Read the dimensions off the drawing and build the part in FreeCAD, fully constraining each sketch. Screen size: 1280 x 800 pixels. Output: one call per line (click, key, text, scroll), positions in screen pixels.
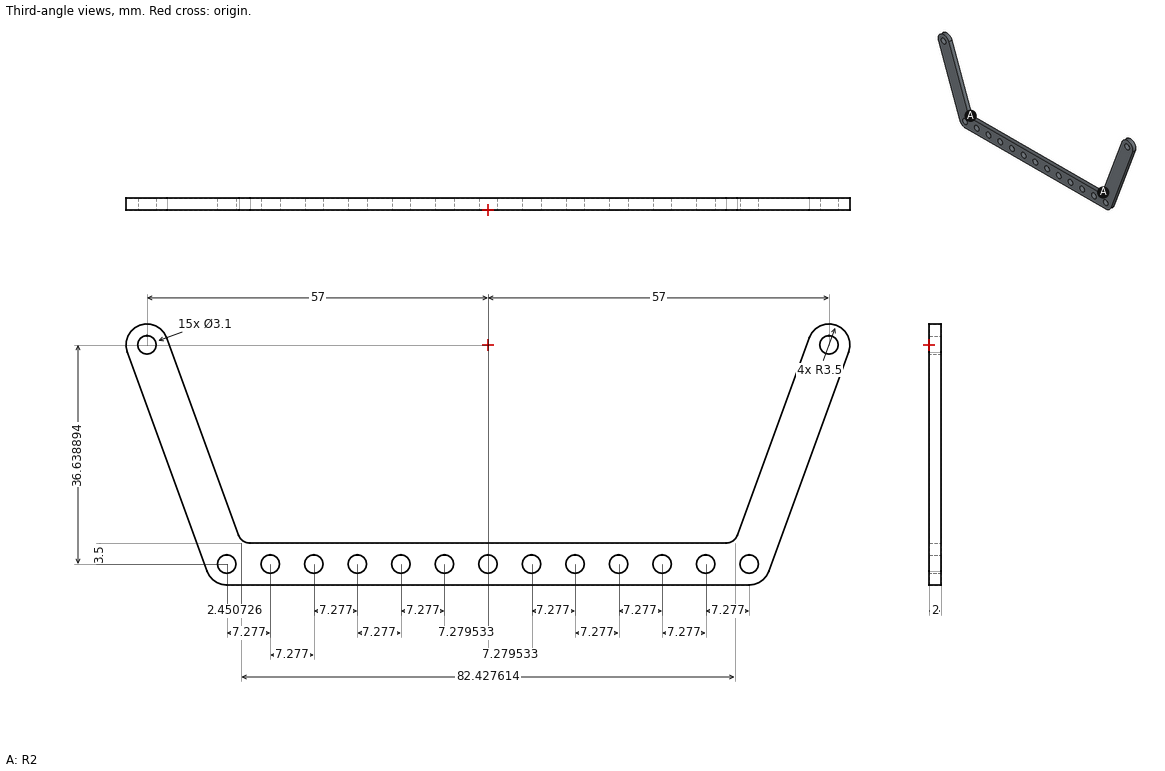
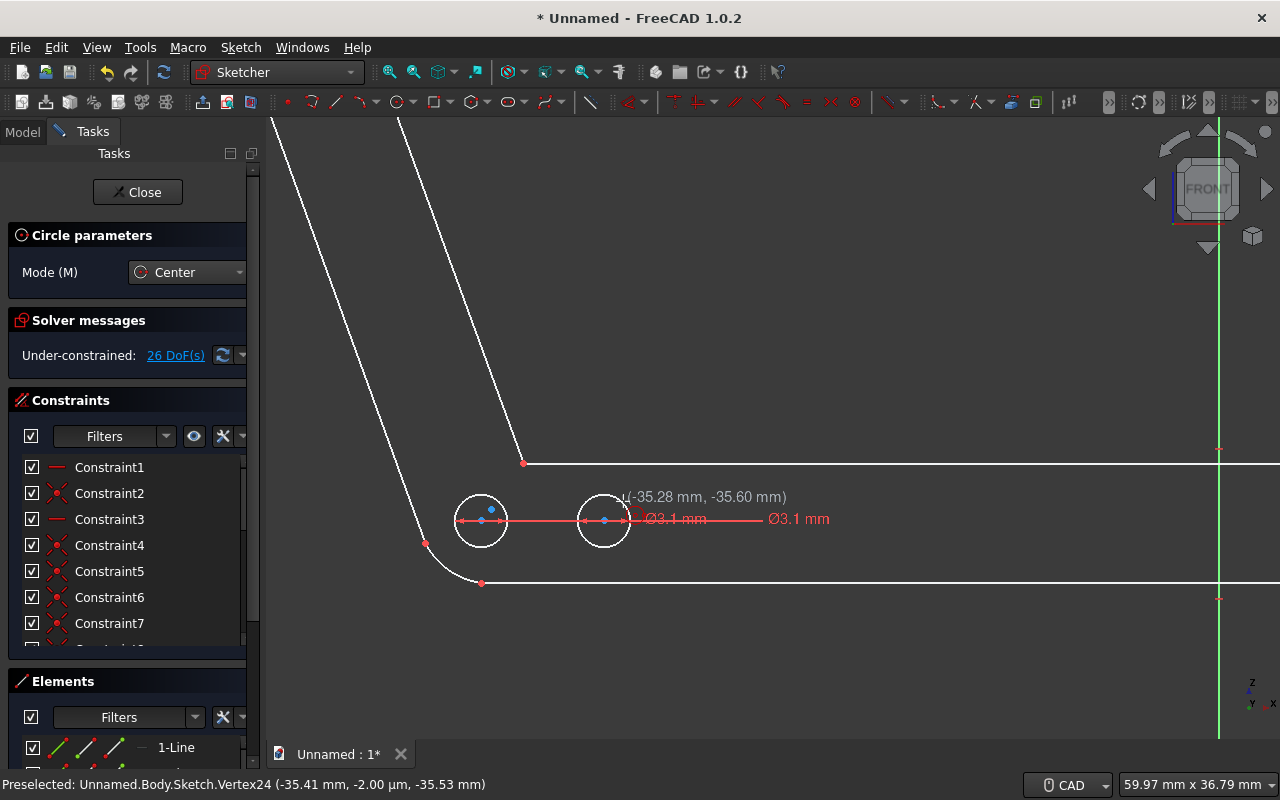
click(727, 520)
move(746, 501)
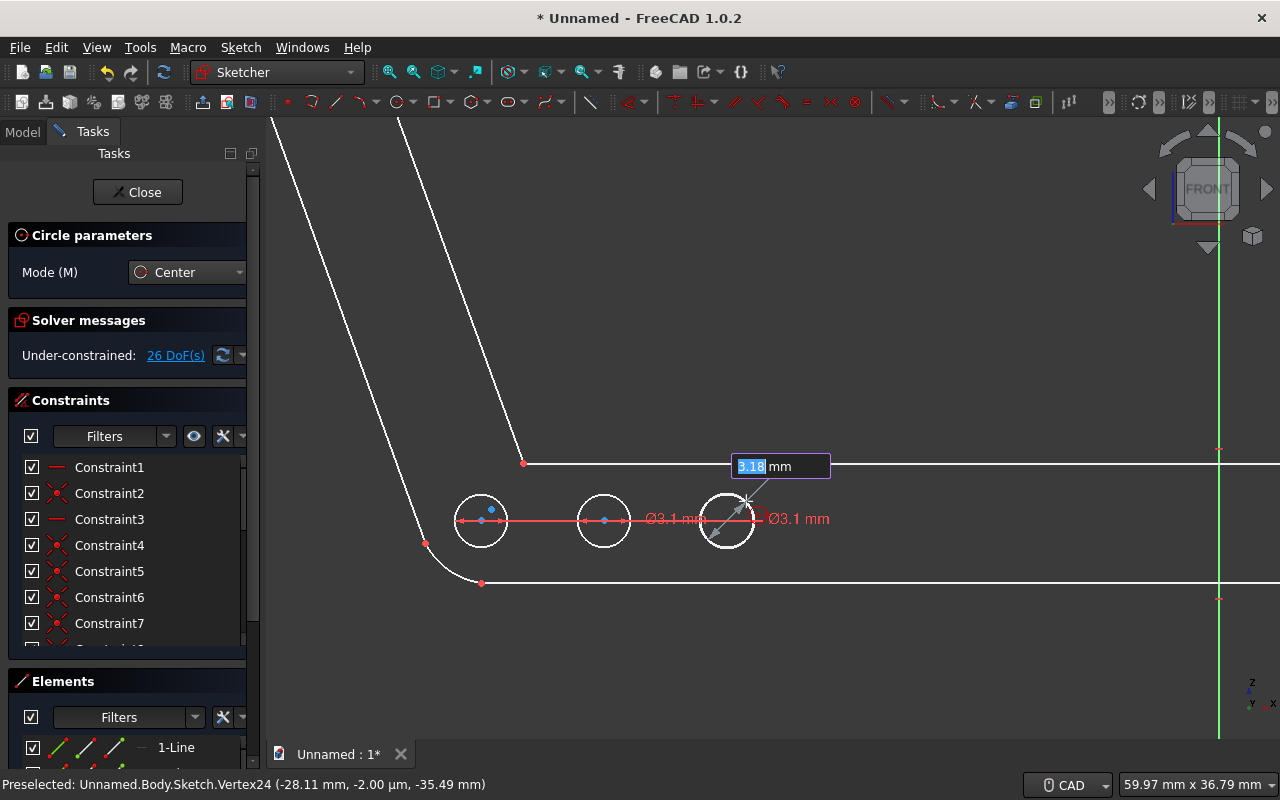
text(3.1)
key(Return)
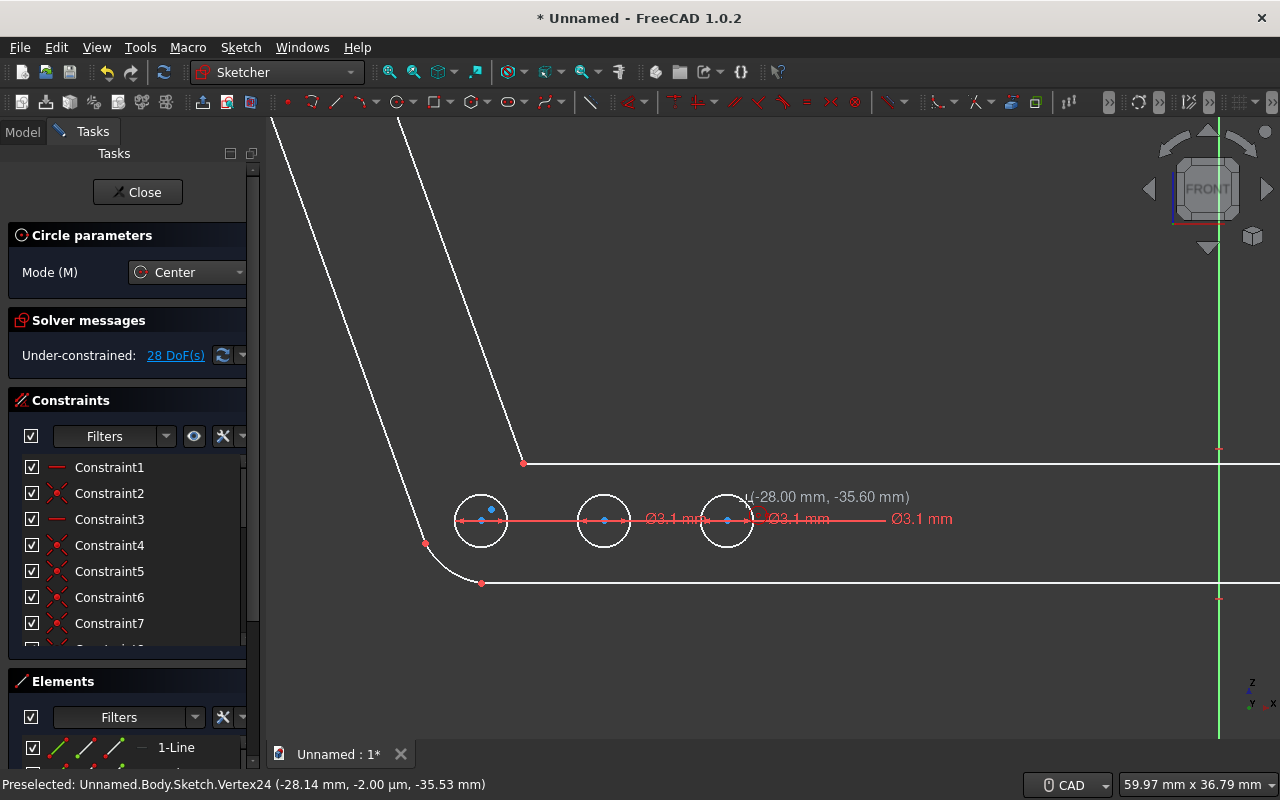
click(850, 520)
move(869, 501)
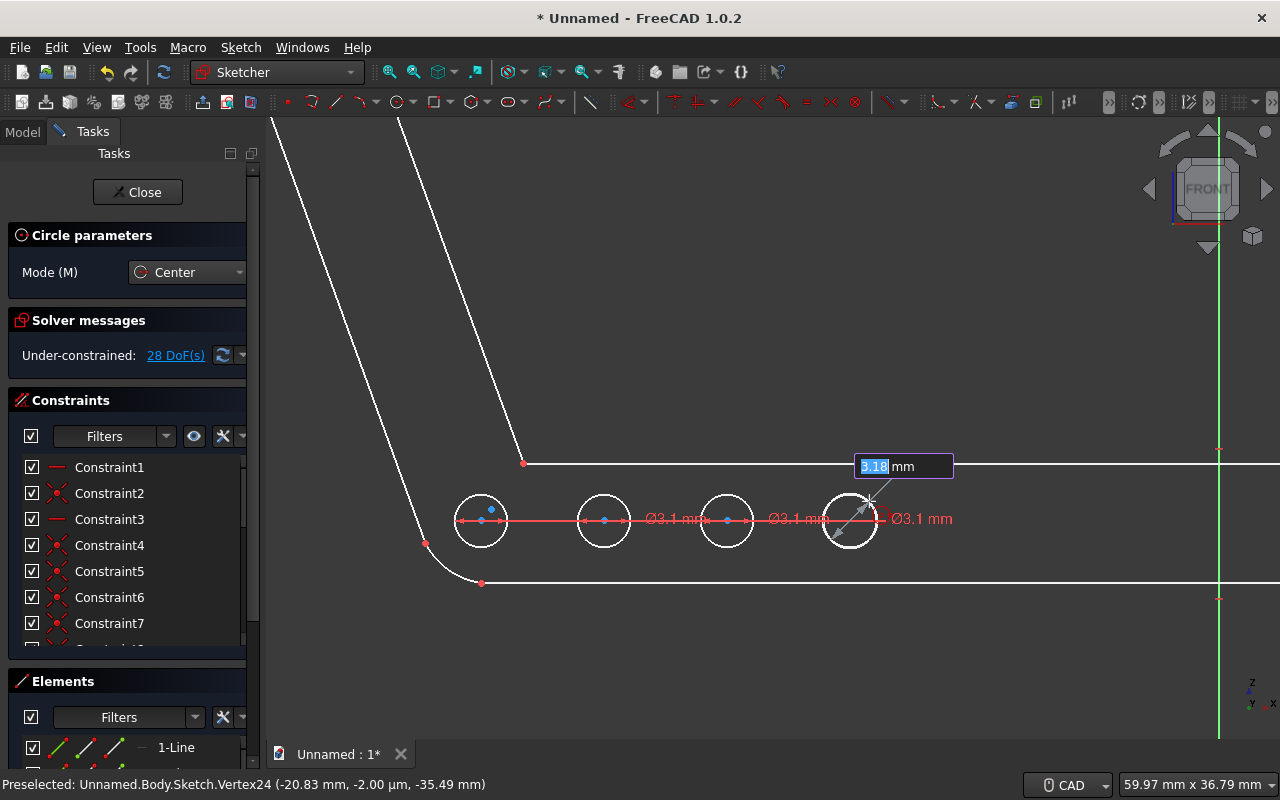
text(3.1)
key(Return)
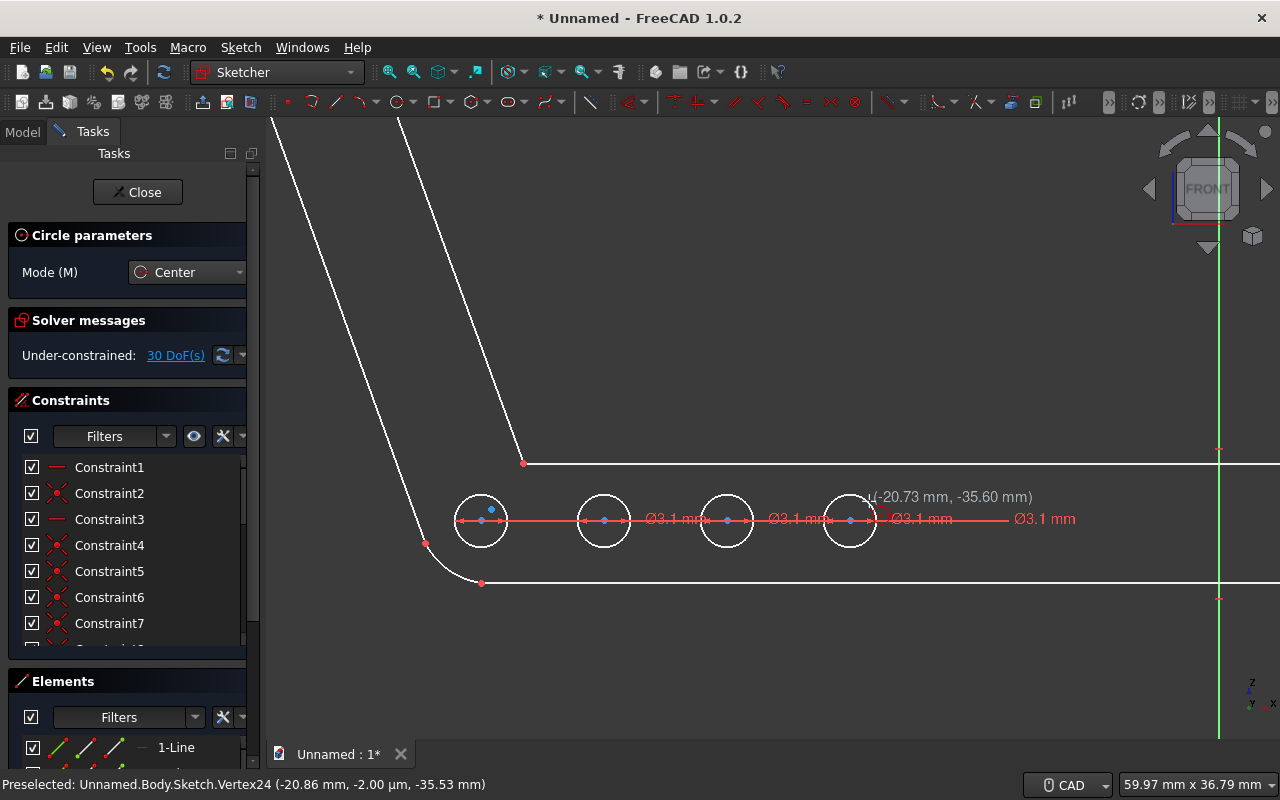
click(973, 520)
move(992, 501)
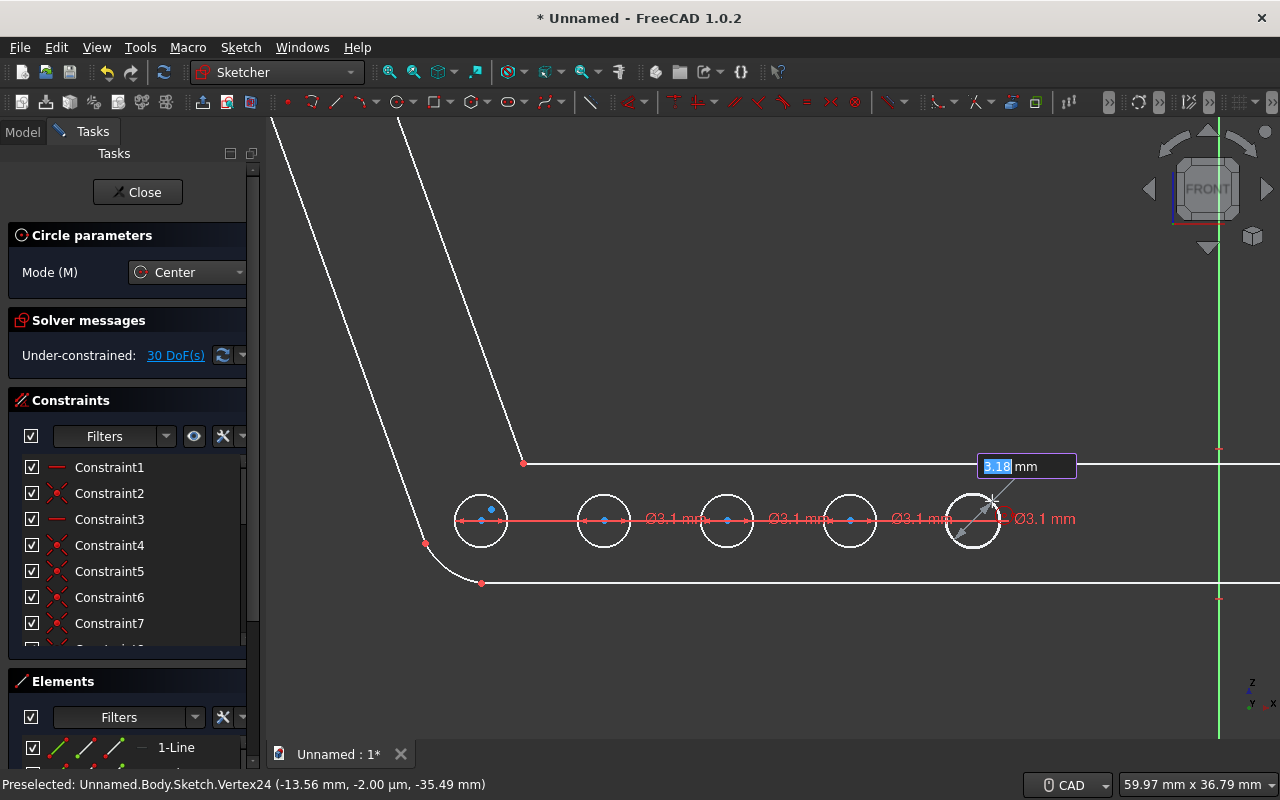
text(3.1)
key(Return)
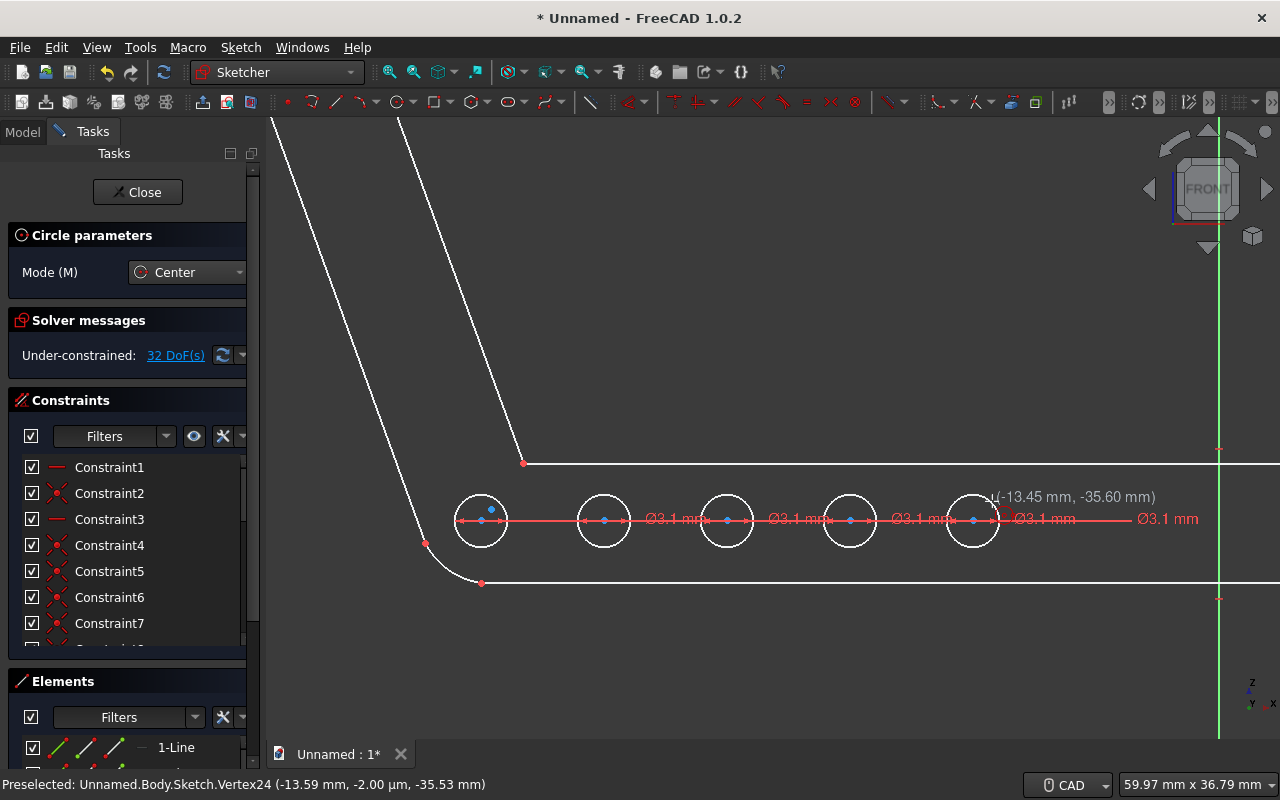
click(1096, 520)
move(1115, 501)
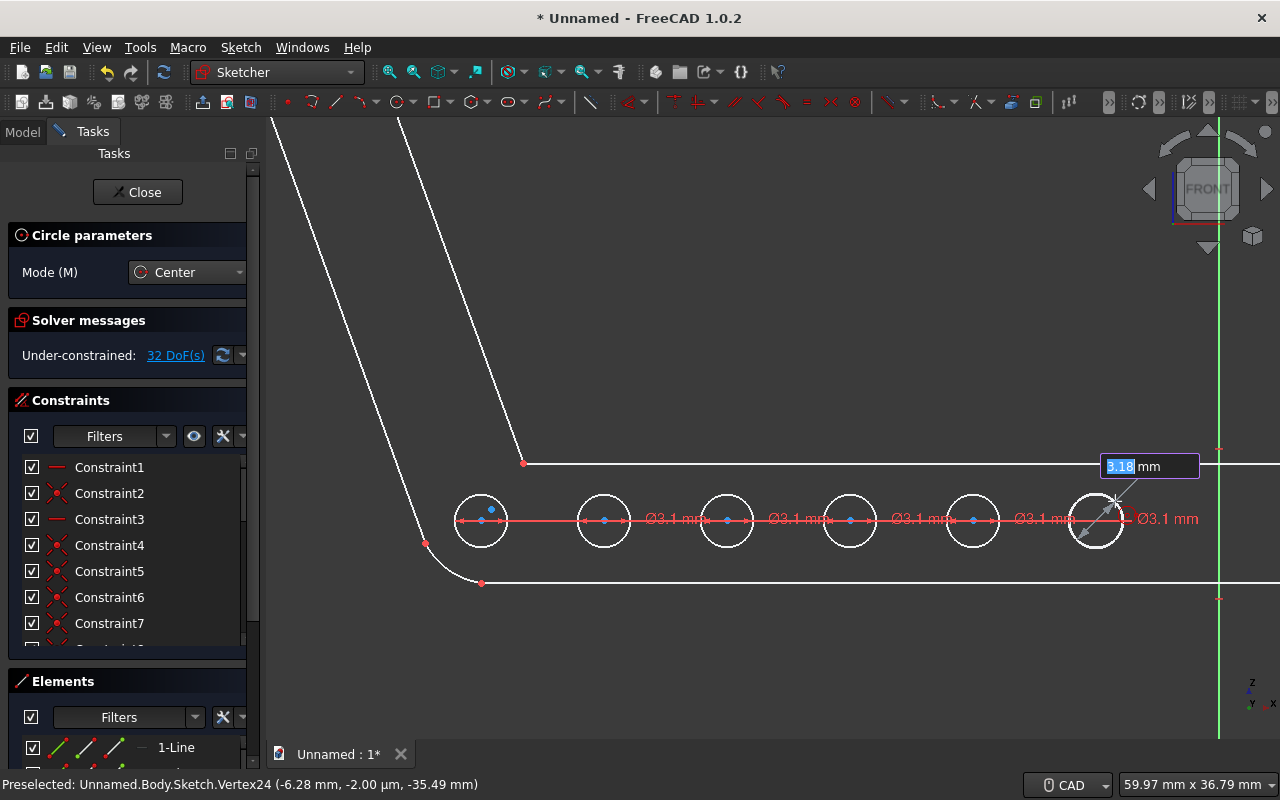
text(3.1)
key(Return)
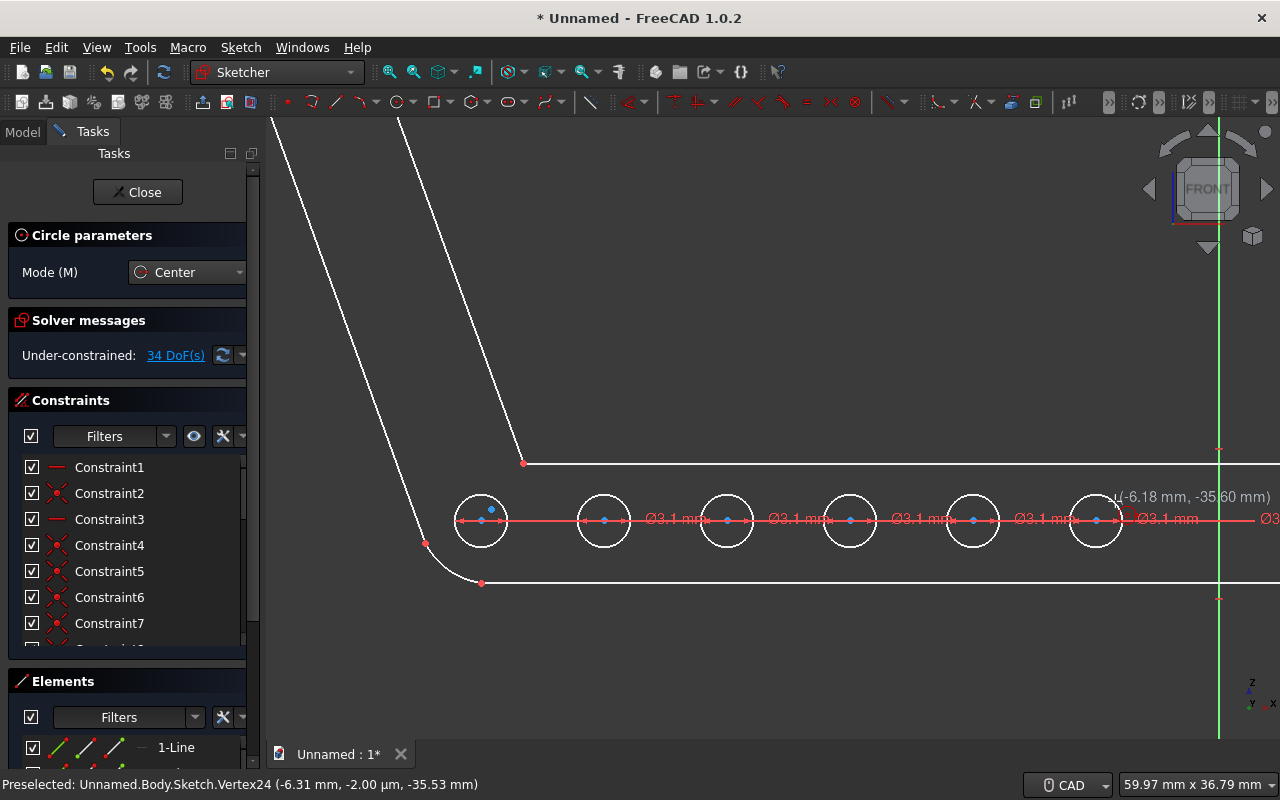
scroll(483, 521, down, 6)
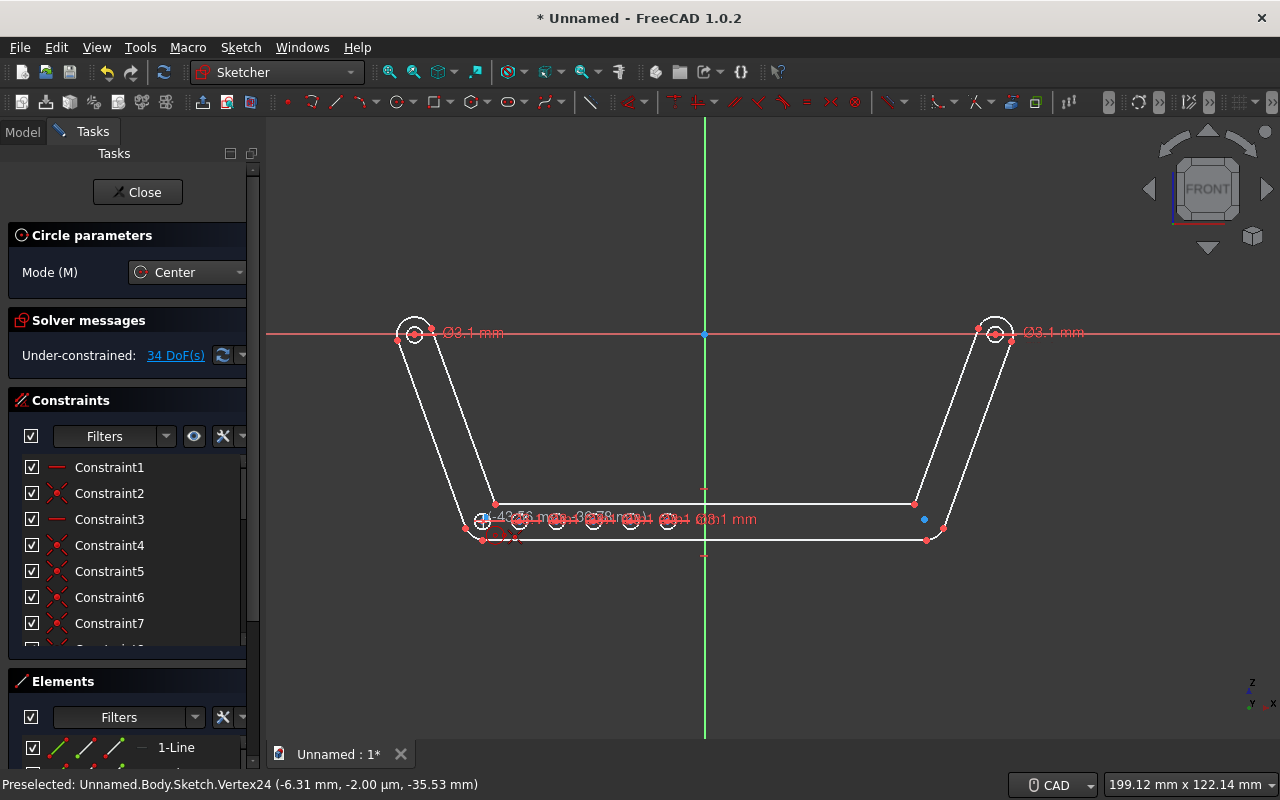
scroll(705, 521, up, 6)